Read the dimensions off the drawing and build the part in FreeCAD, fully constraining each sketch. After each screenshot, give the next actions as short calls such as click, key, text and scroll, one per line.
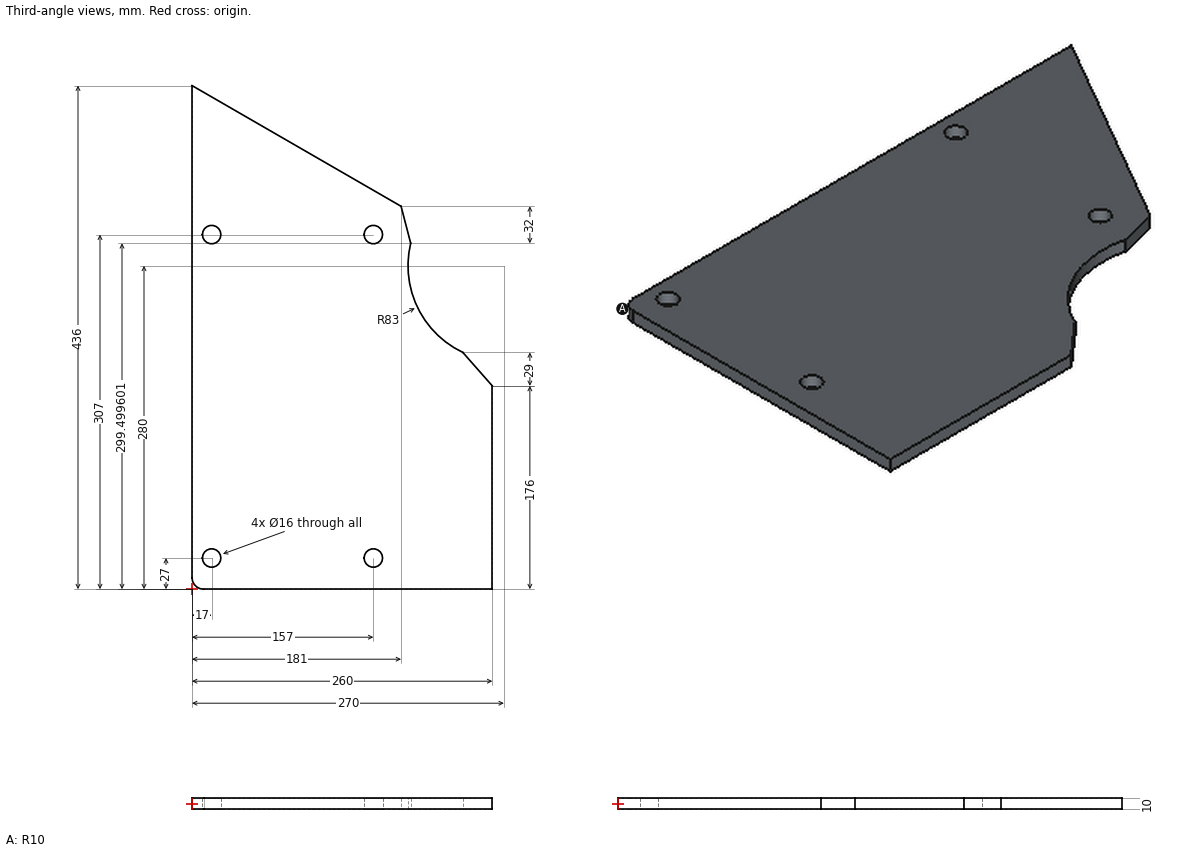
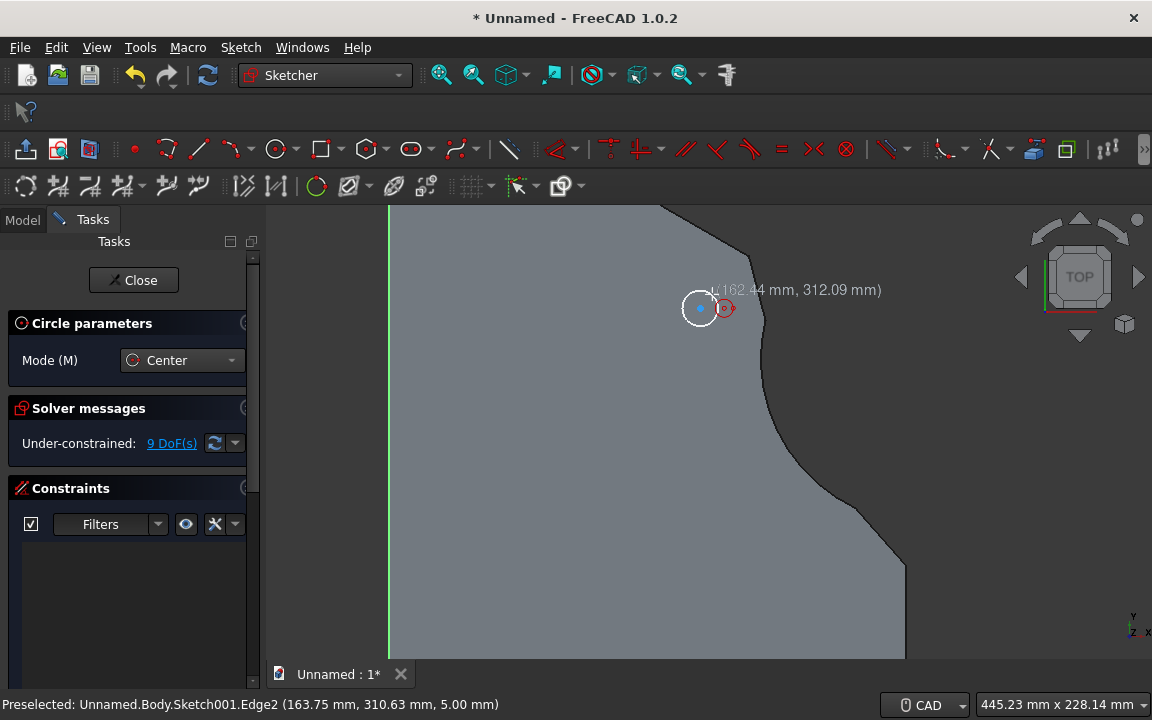
scroll(423, 305, up, 2)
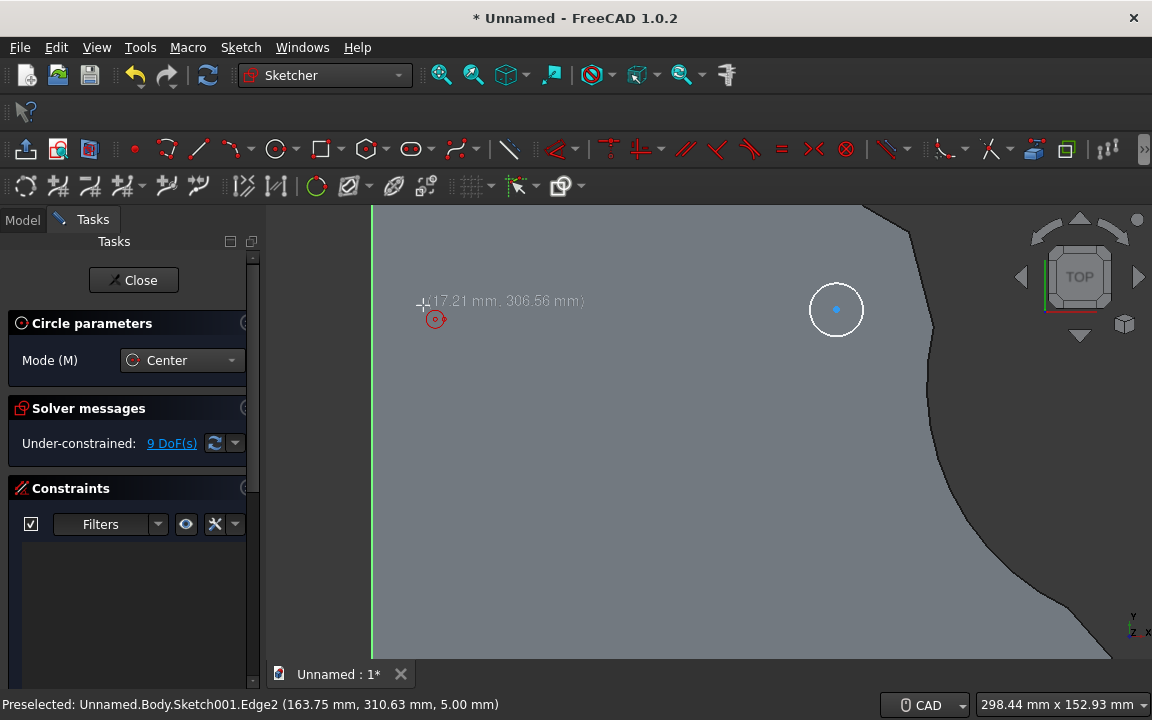
scroll(651, 295, down, 6)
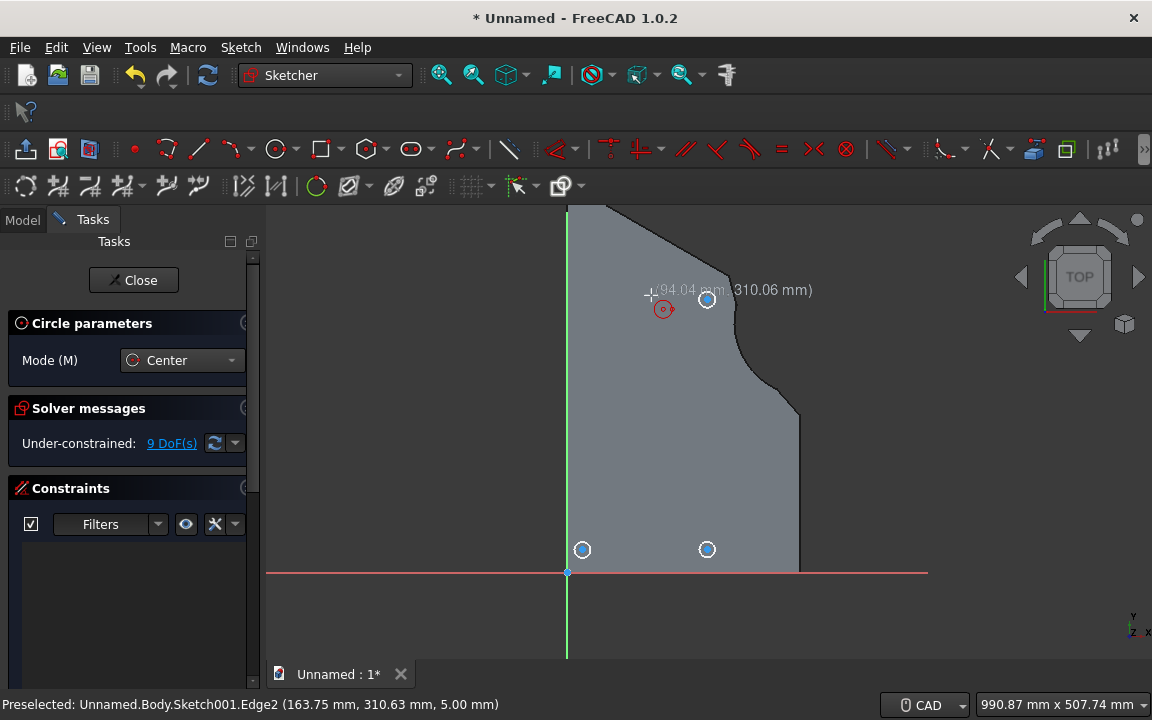
click(582, 298)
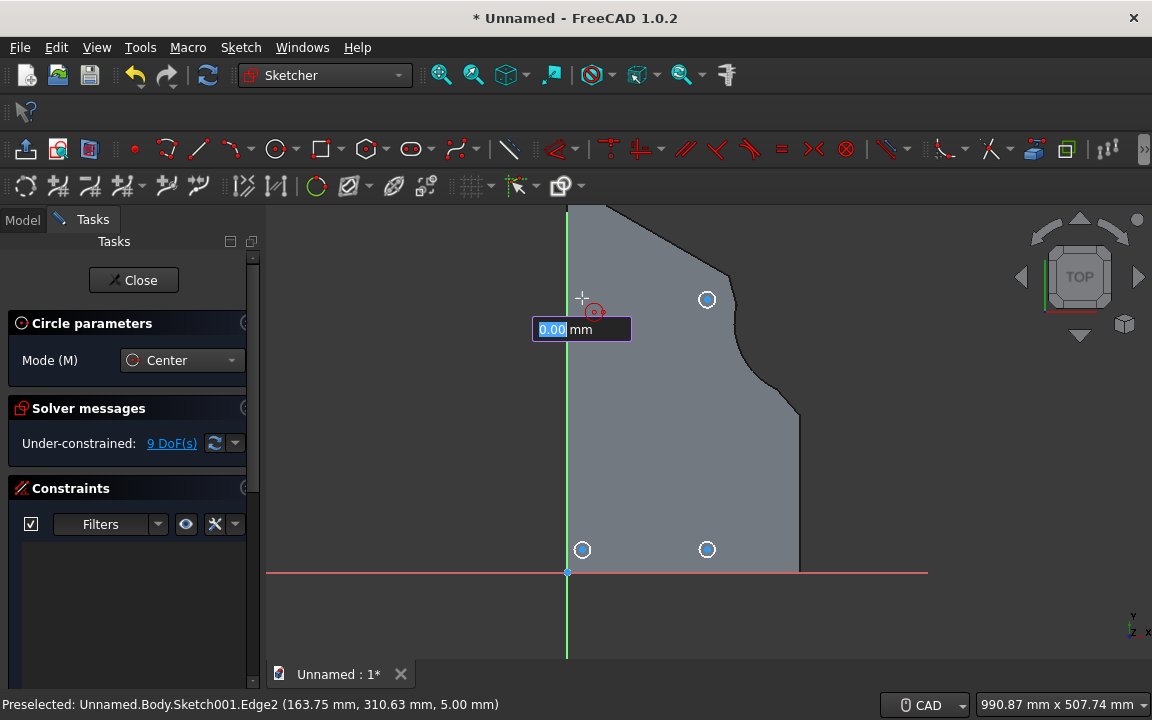
scroll(587, 293, up, 4)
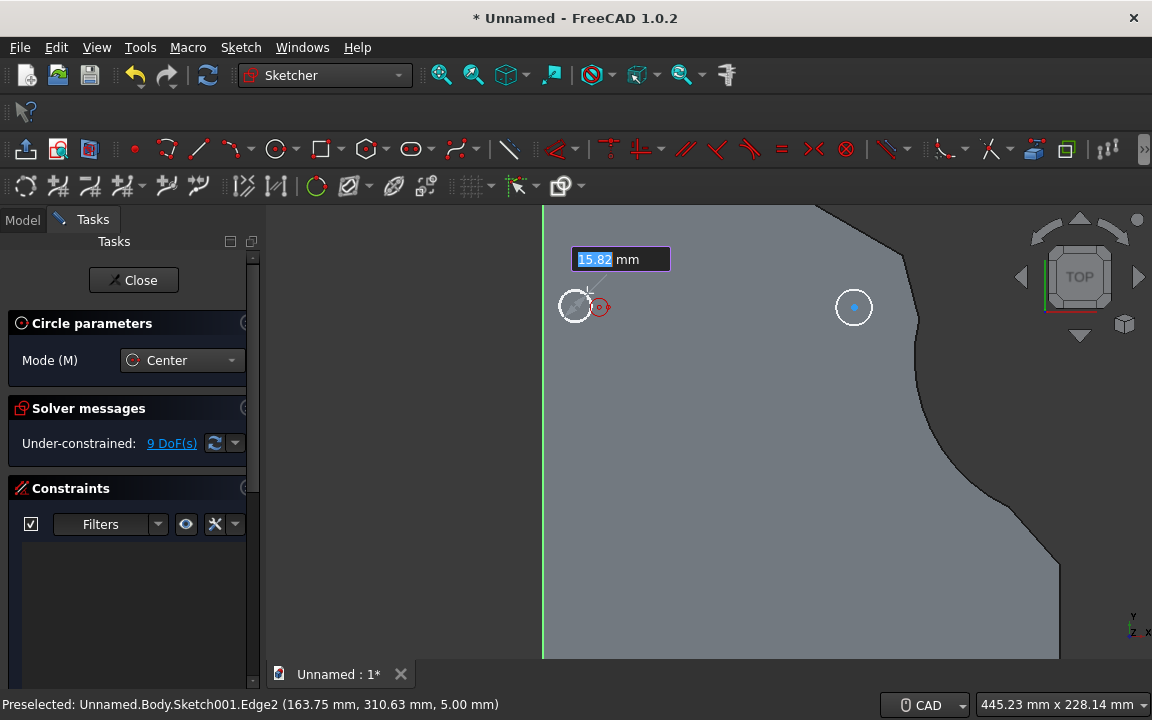
click(588, 293)
key(Escape)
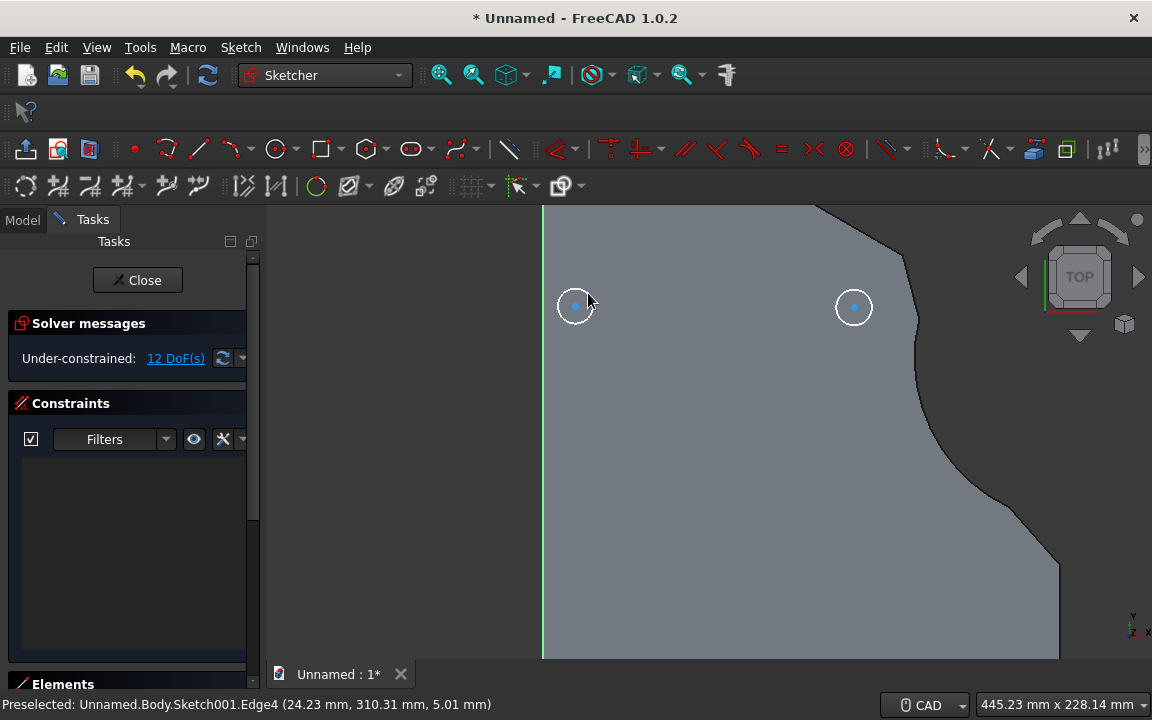
scroll(586, 293, down, 4)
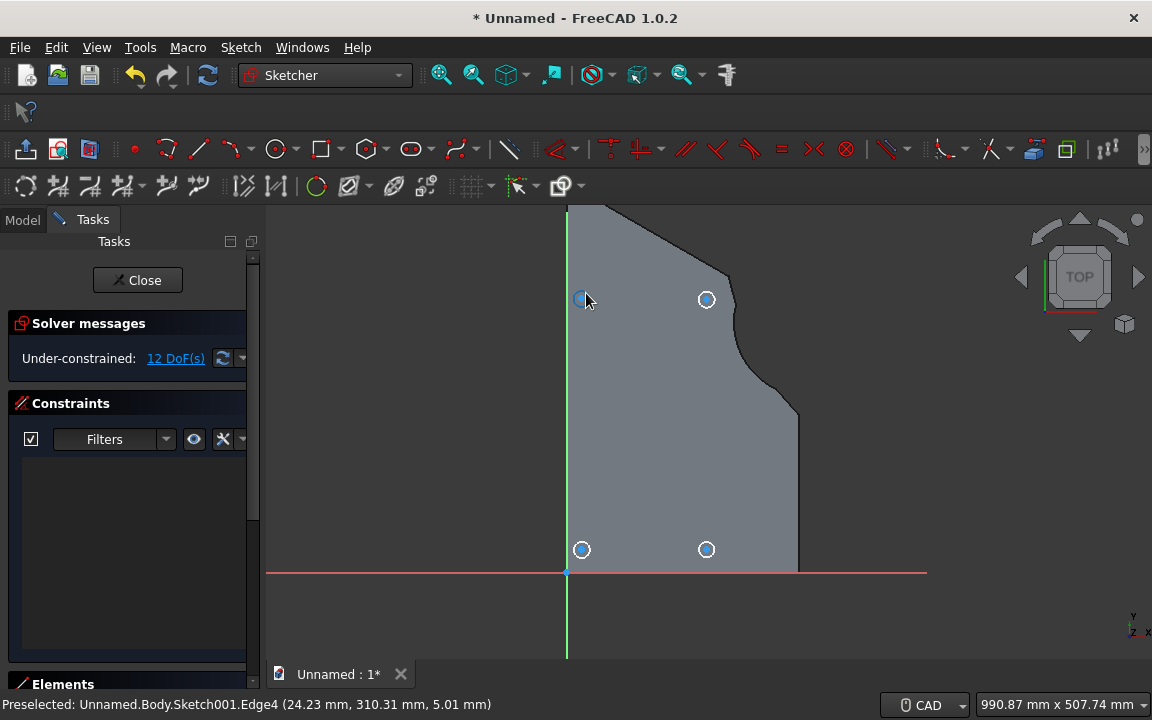
scroll(588, 544, up, 3)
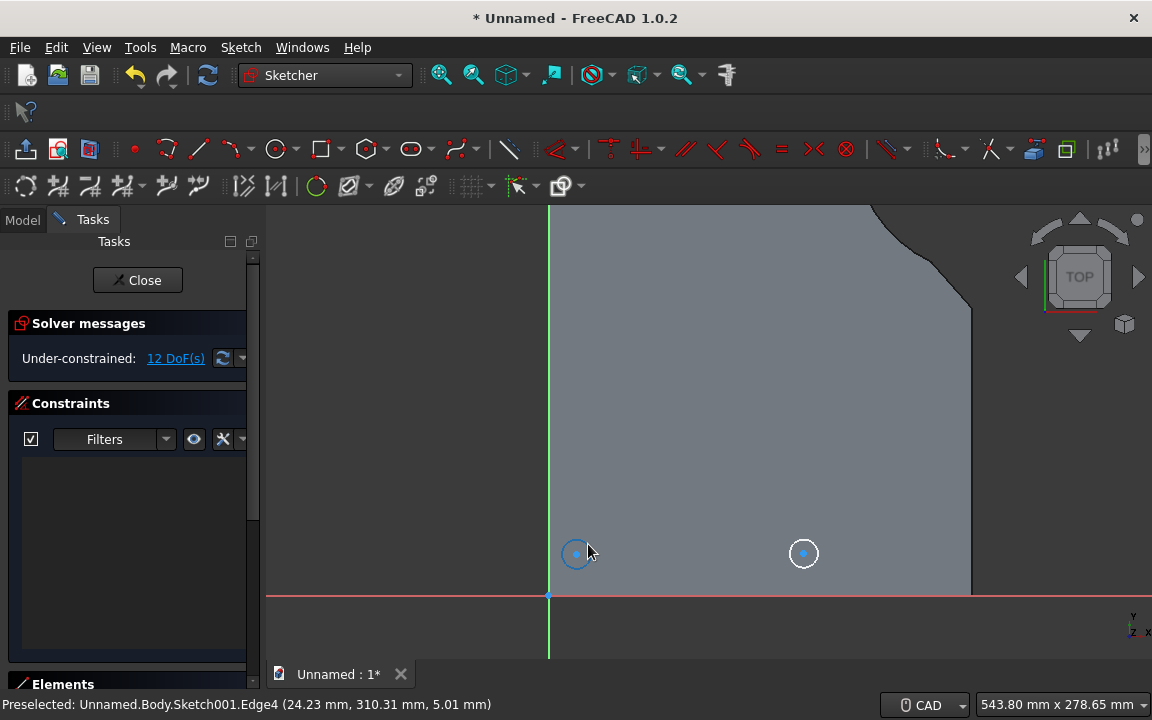
click(587, 544)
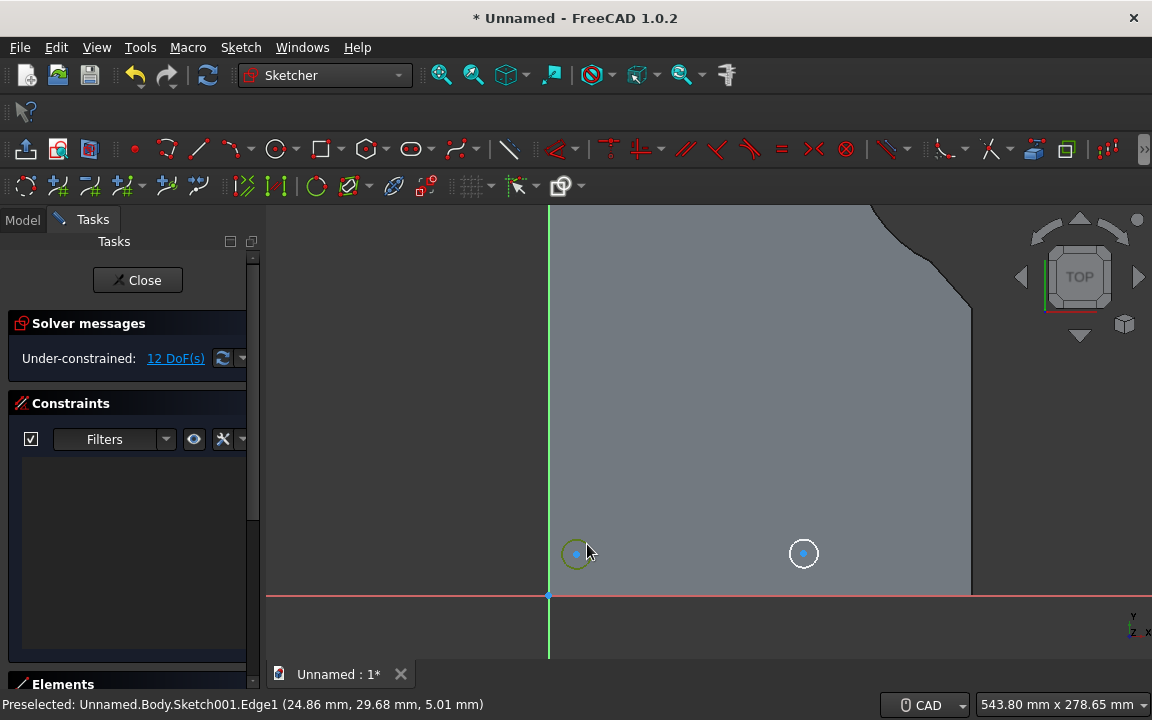
click(814, 544)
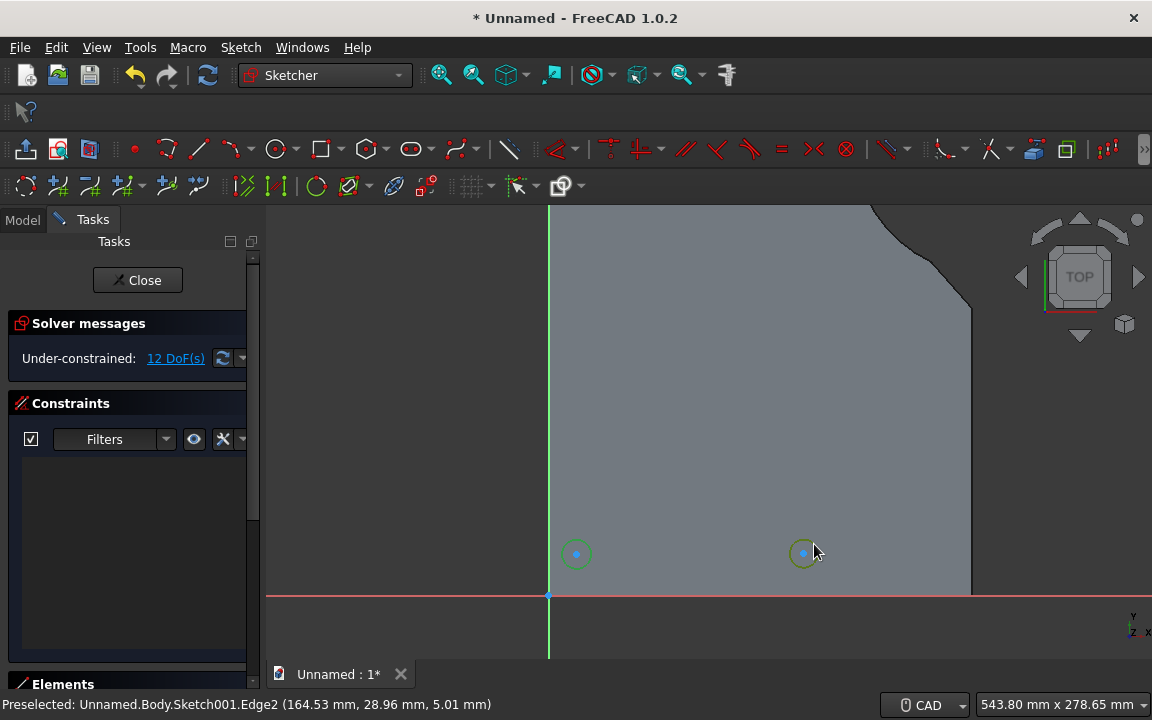
scroll(589, 545, down, 3)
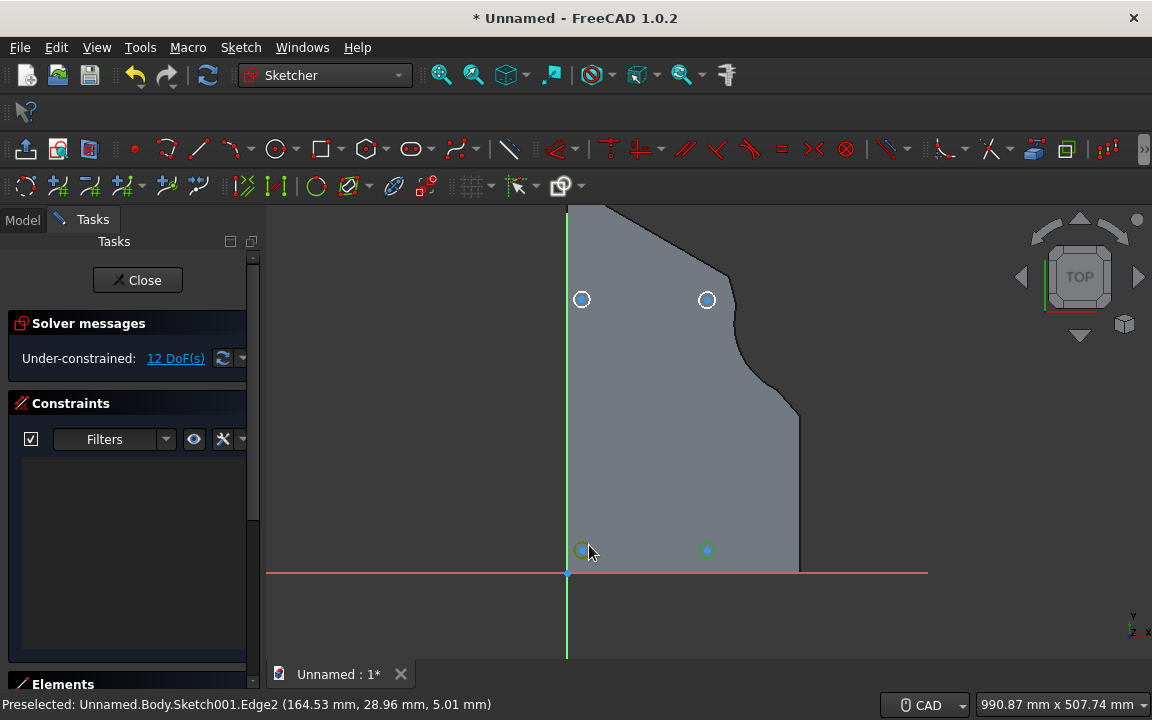
scroll(713, 294, up, 3)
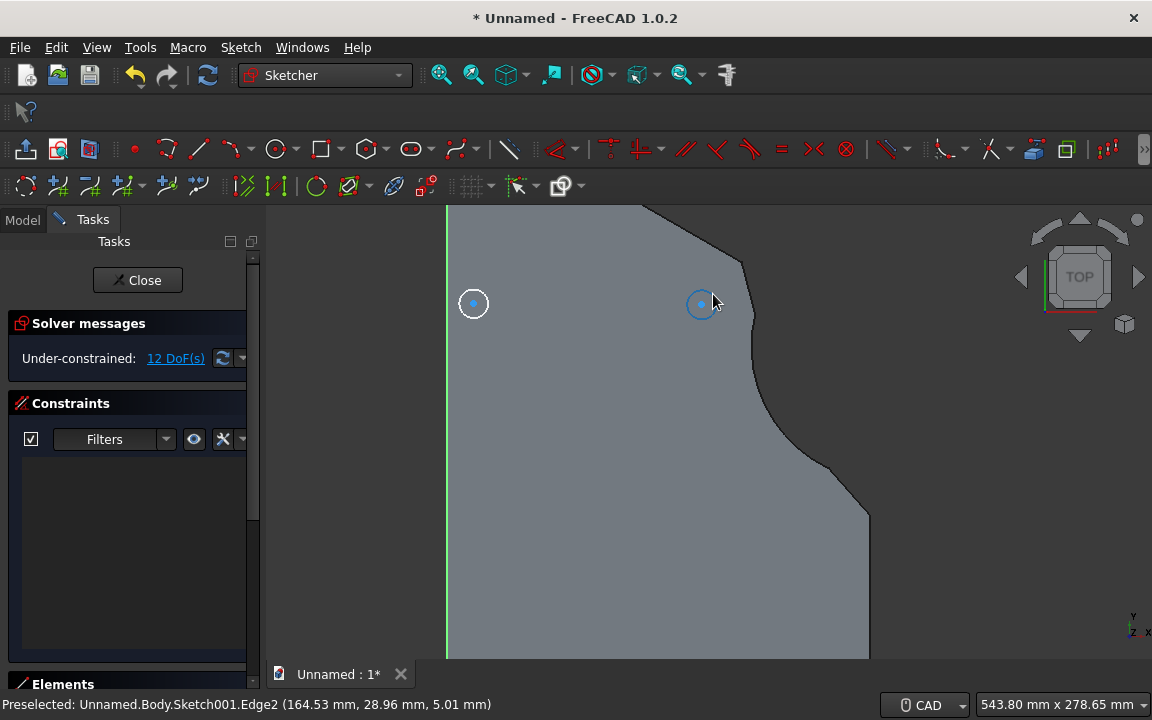
click(712, 295)